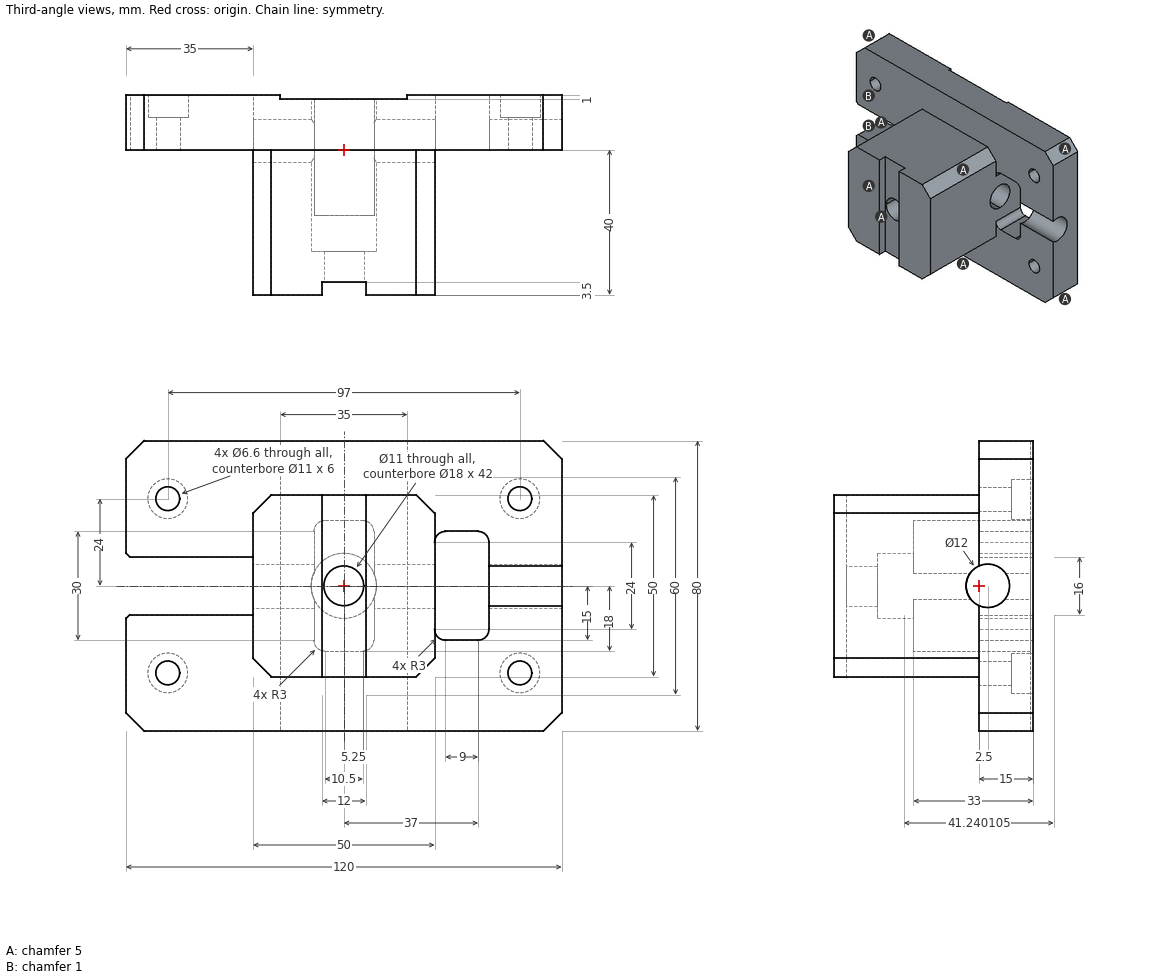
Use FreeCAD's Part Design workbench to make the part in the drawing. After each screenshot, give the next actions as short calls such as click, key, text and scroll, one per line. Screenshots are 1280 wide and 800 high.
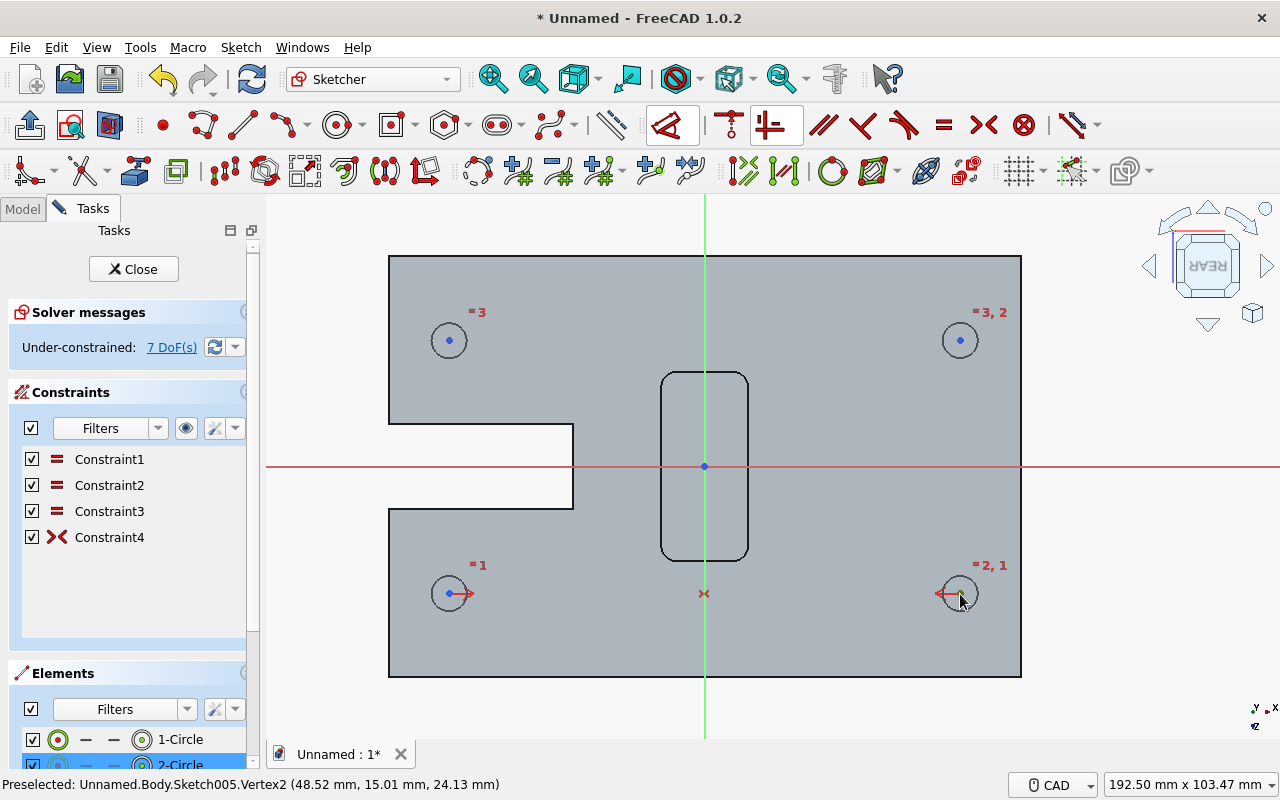
click(960, 340)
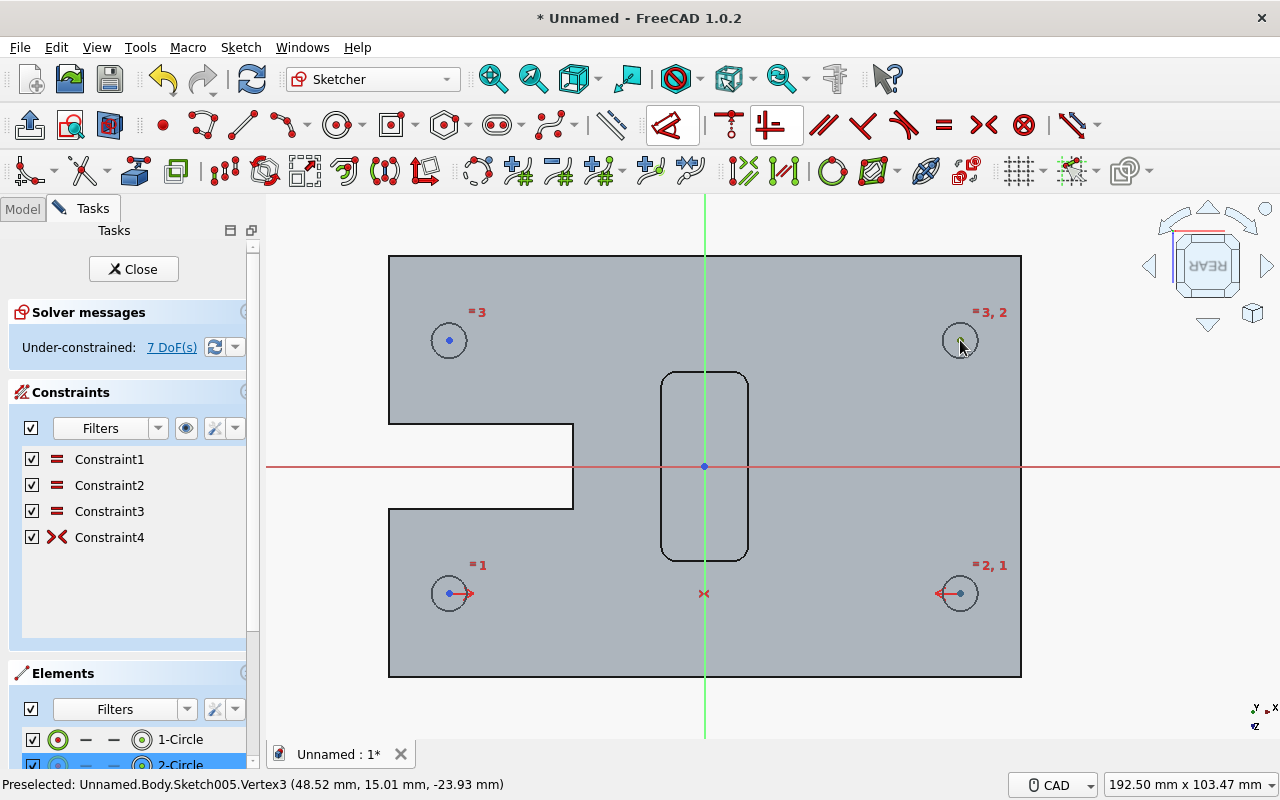
click(353, 466)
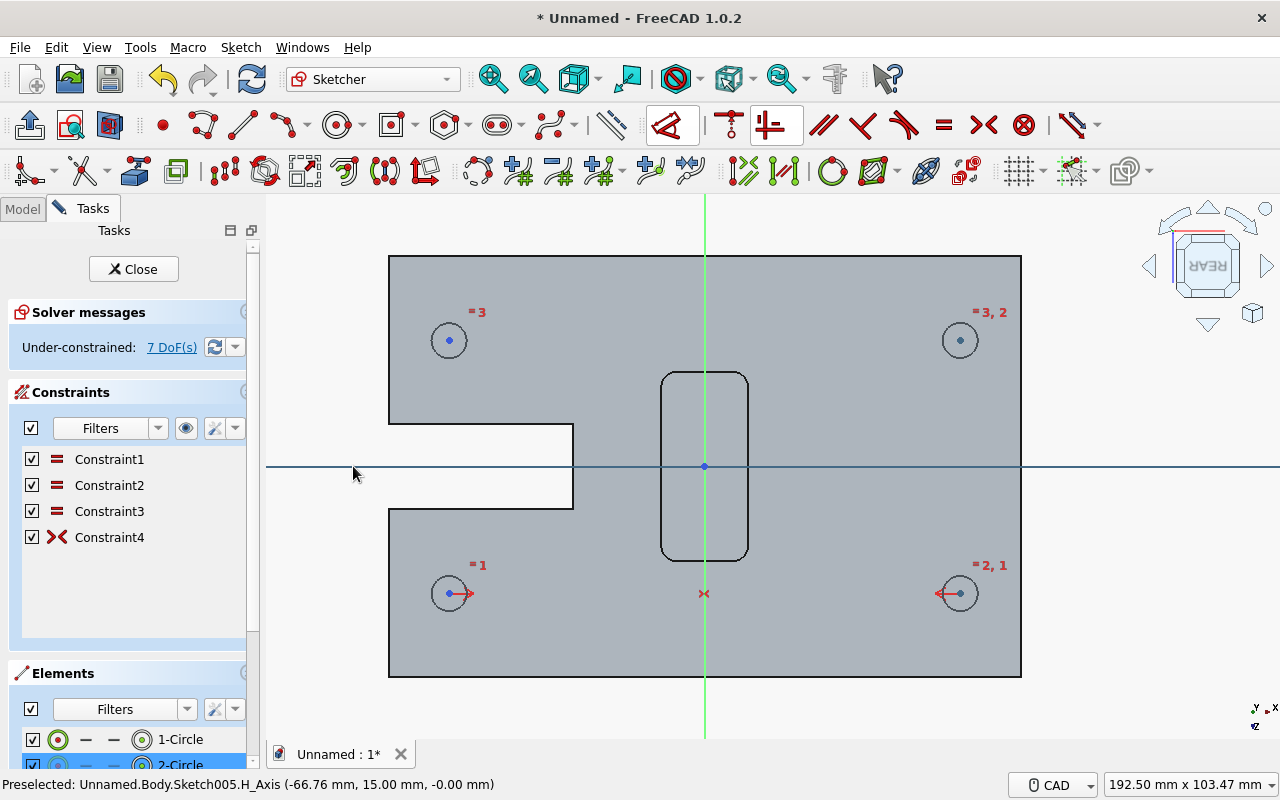
click(984, 126)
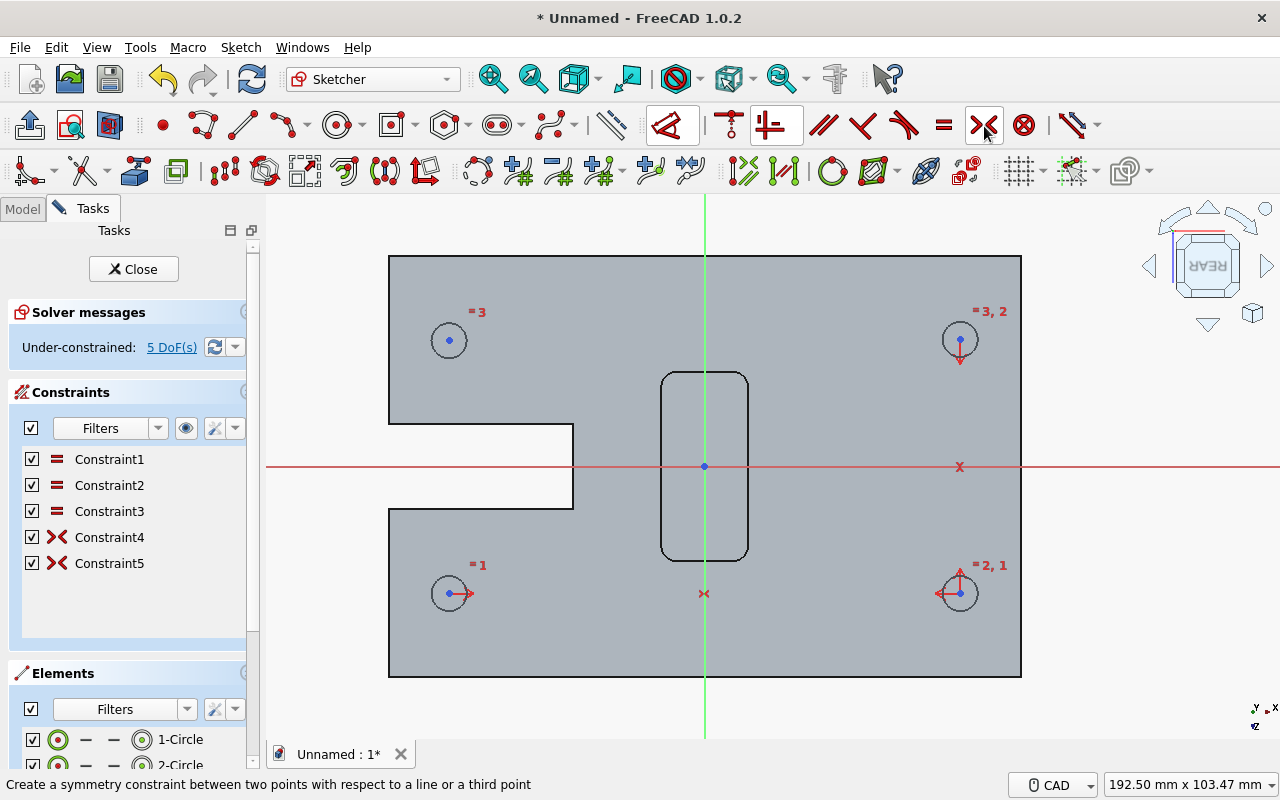
click(449, 594)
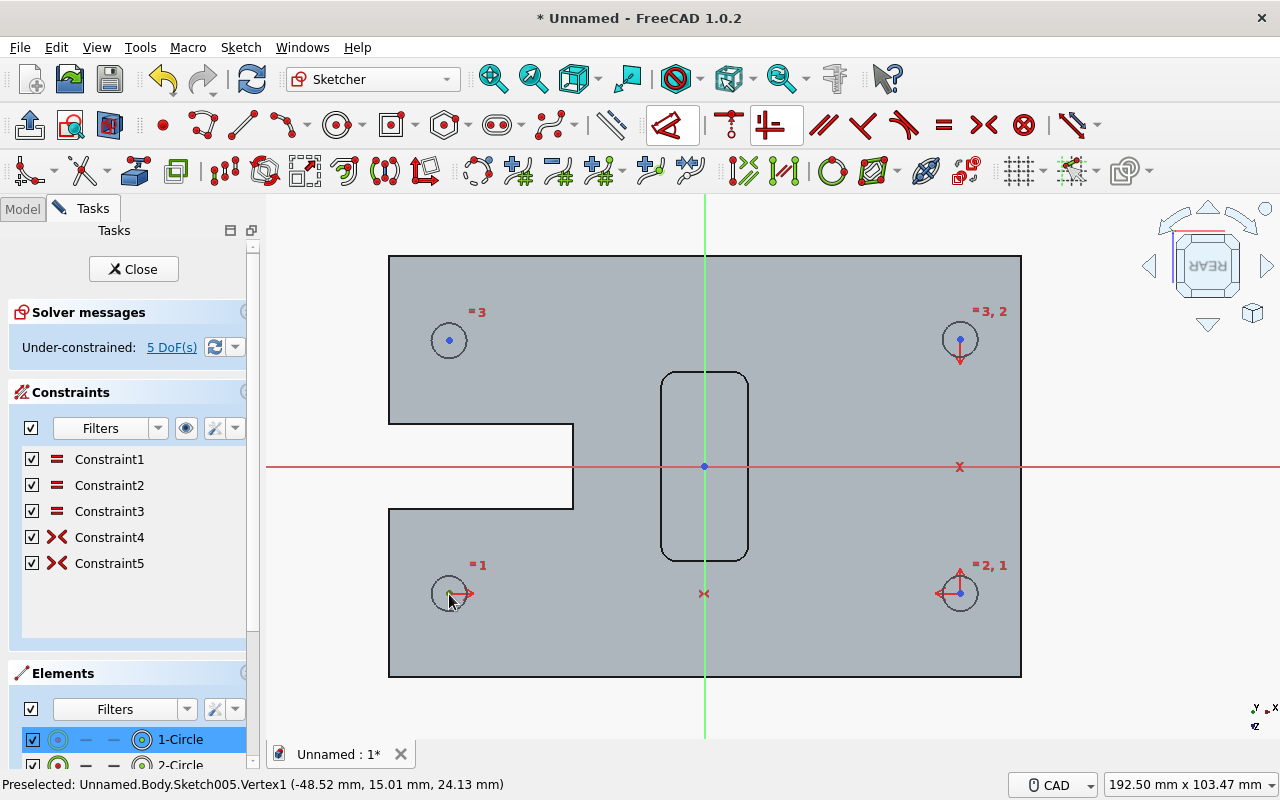
click(449, 341)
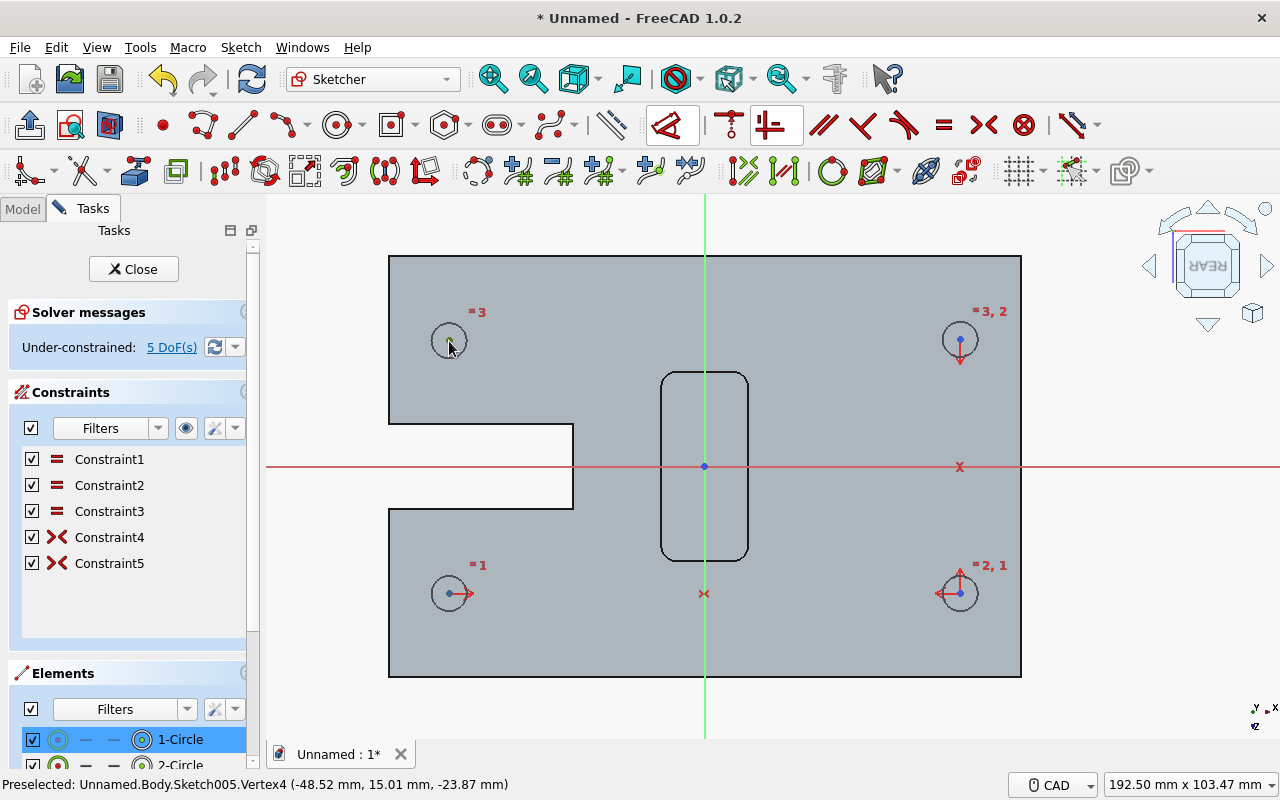
click(353, 466)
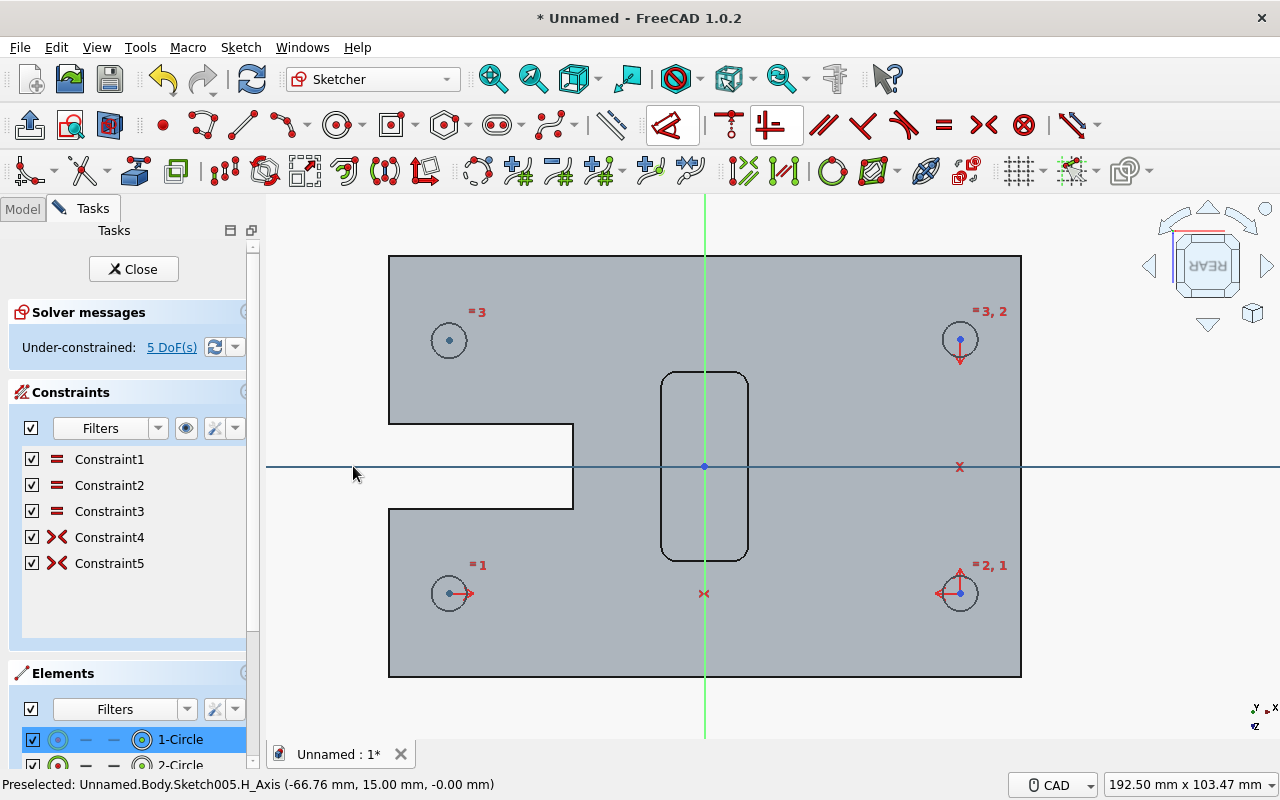
click(984, 126)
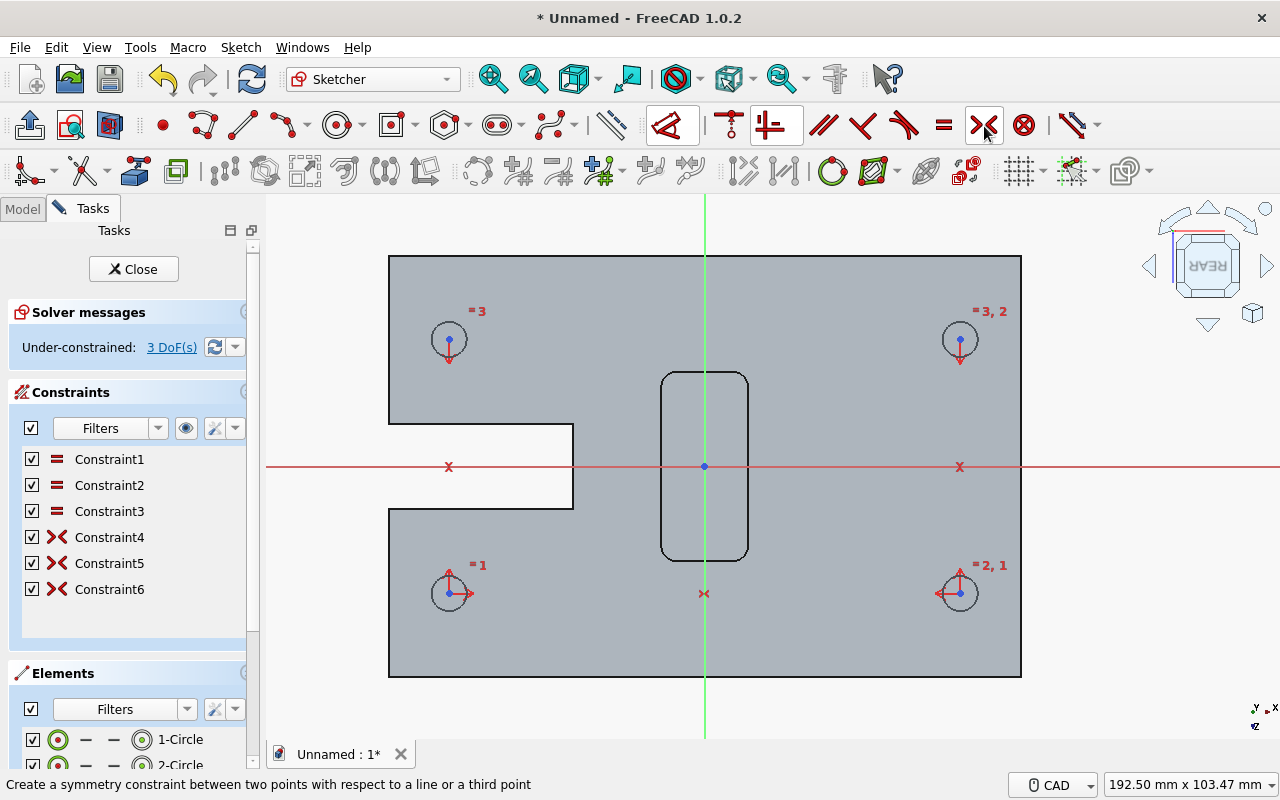
click(461, 581)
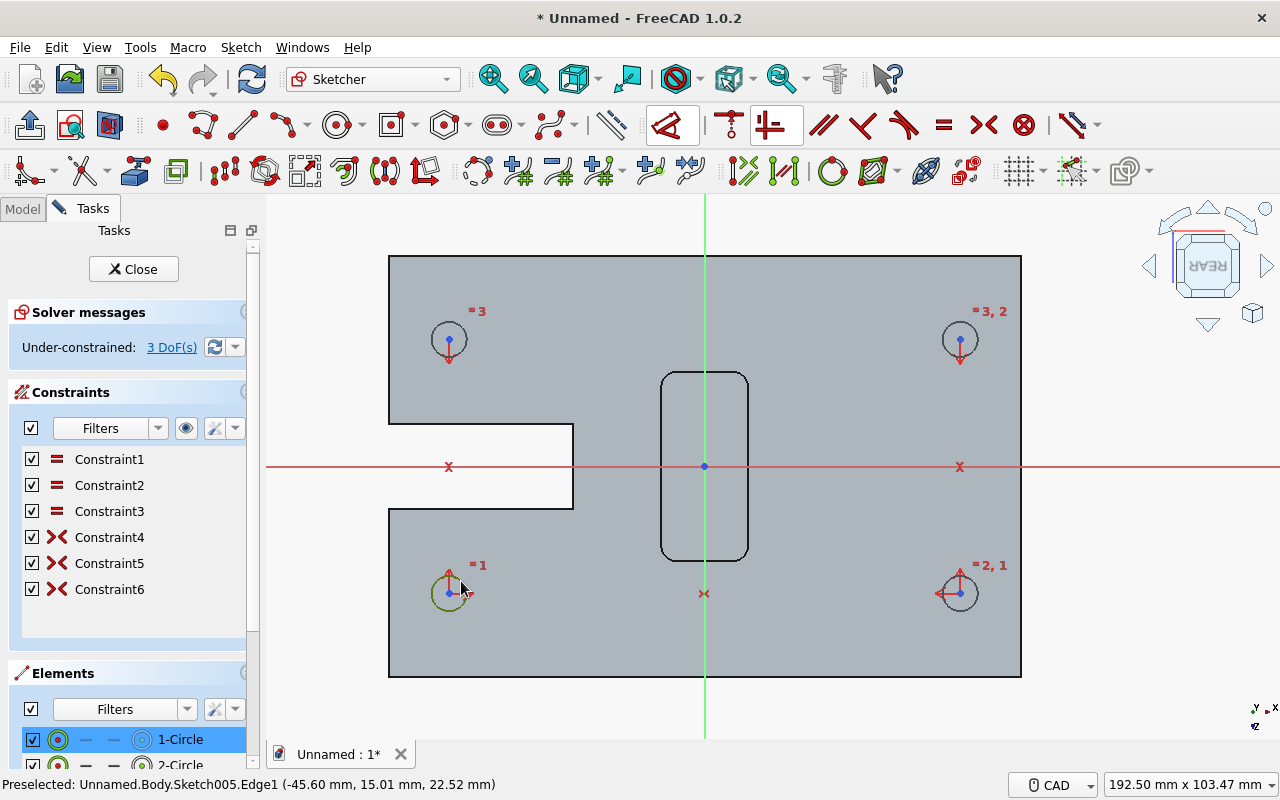
click(694, 126)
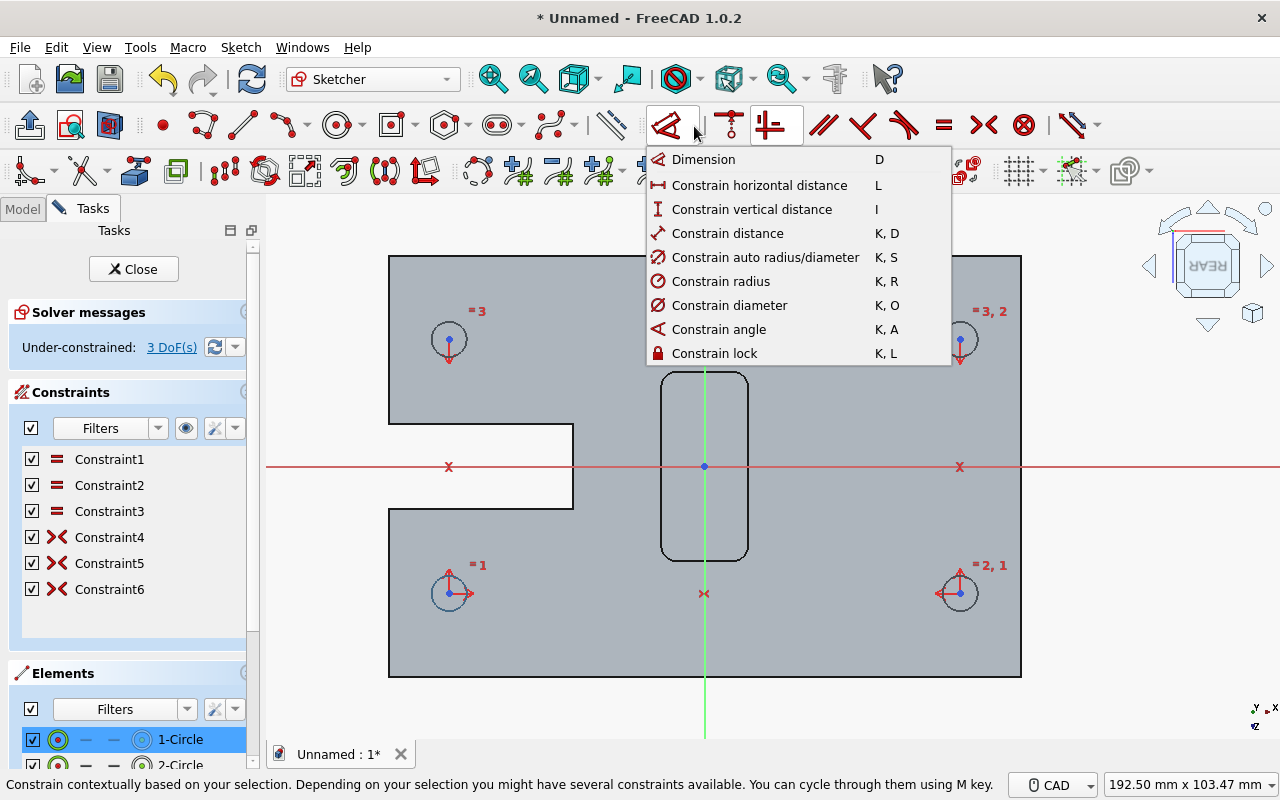
click(799, 305)